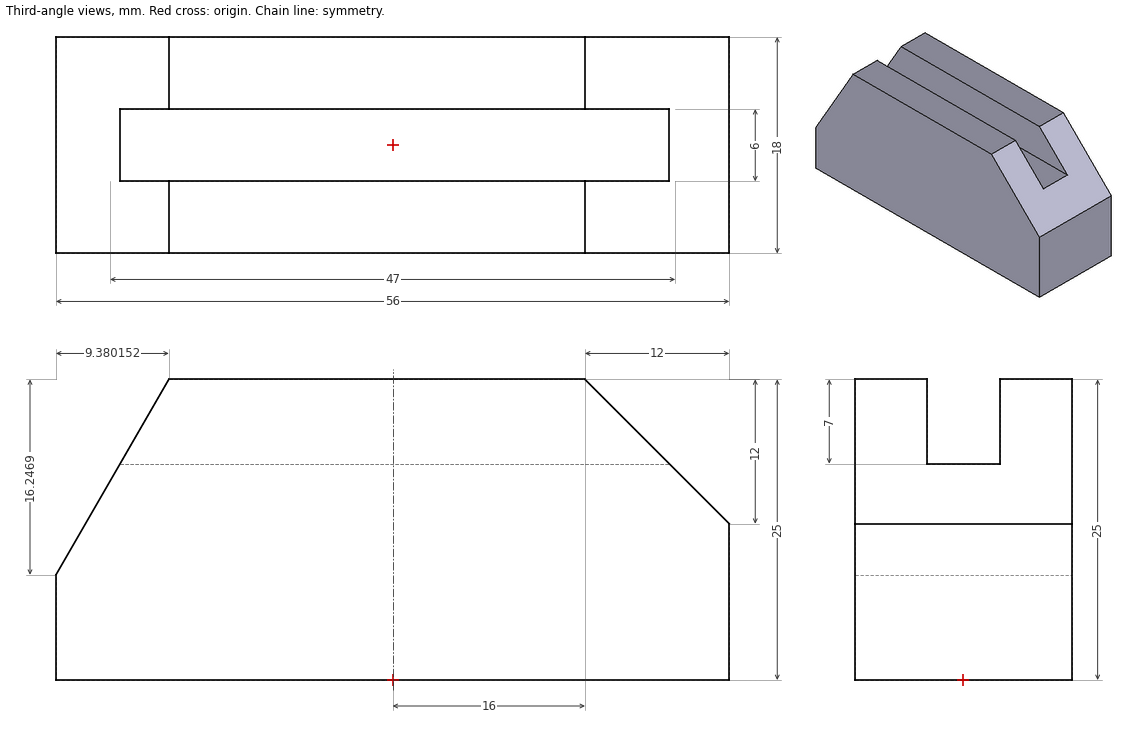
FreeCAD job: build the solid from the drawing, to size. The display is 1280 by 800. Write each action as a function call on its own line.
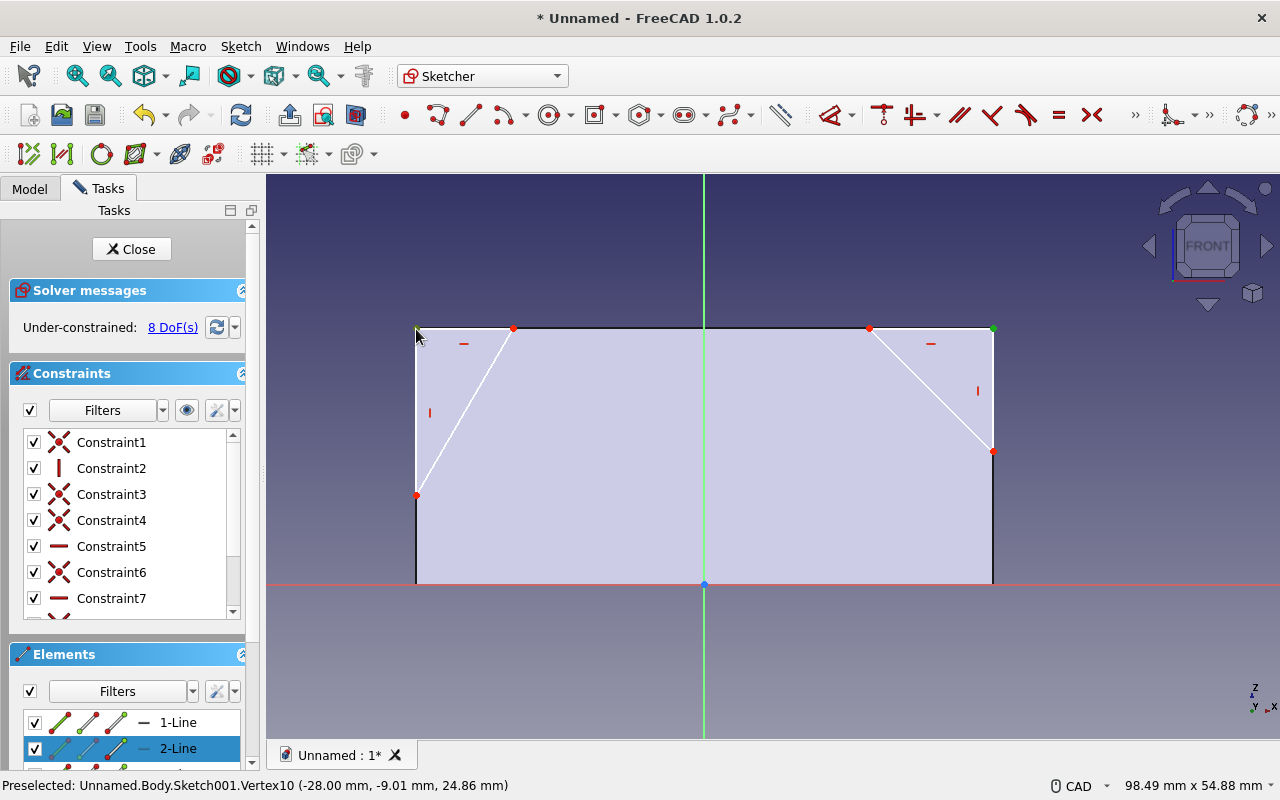
click(704, 675)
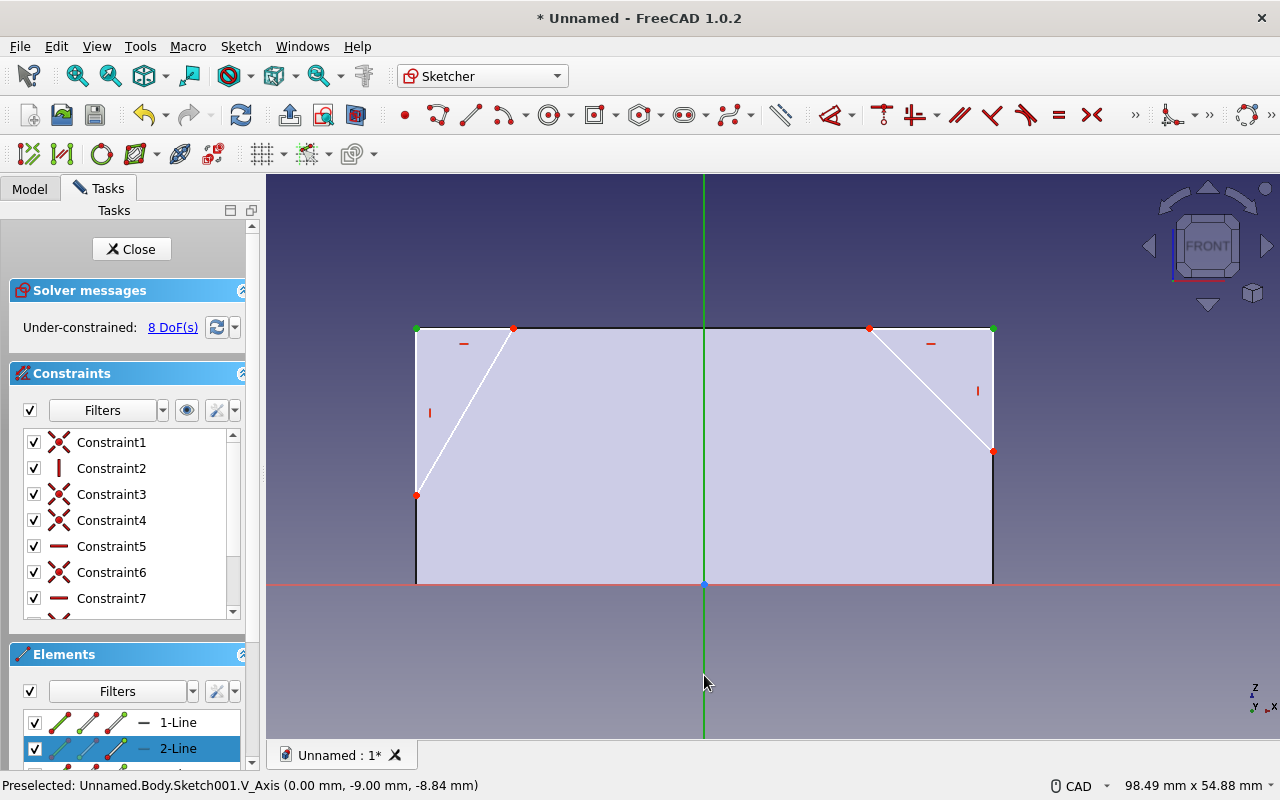
click(1092, 116)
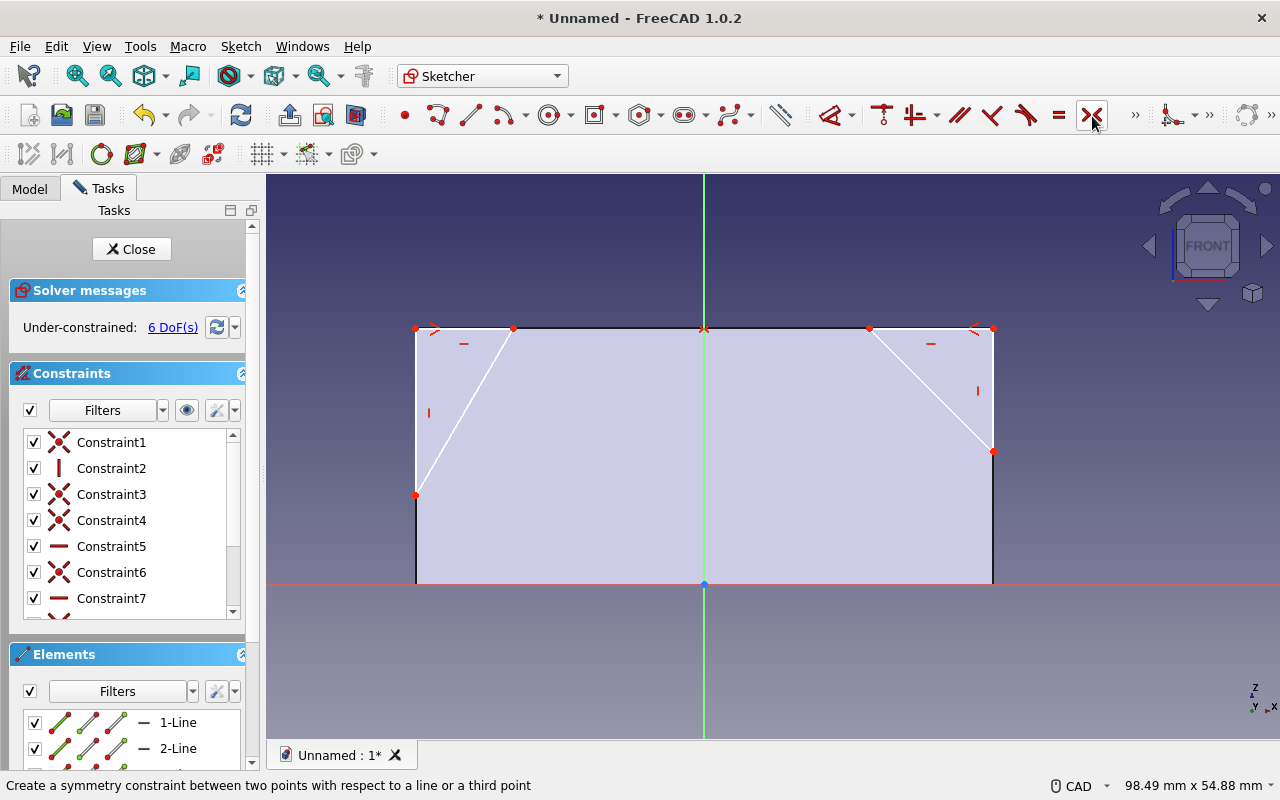
click(830, 116)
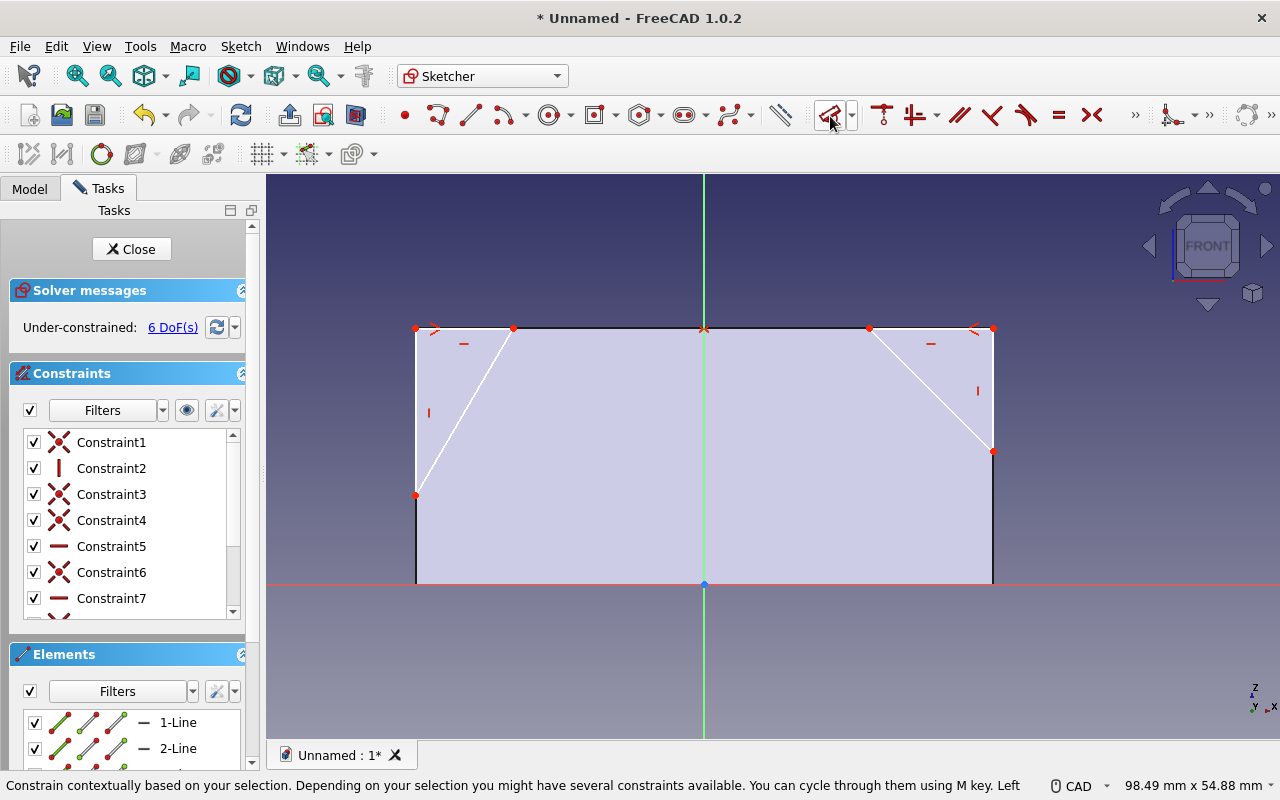
click(993, 415)
click(1027, 390)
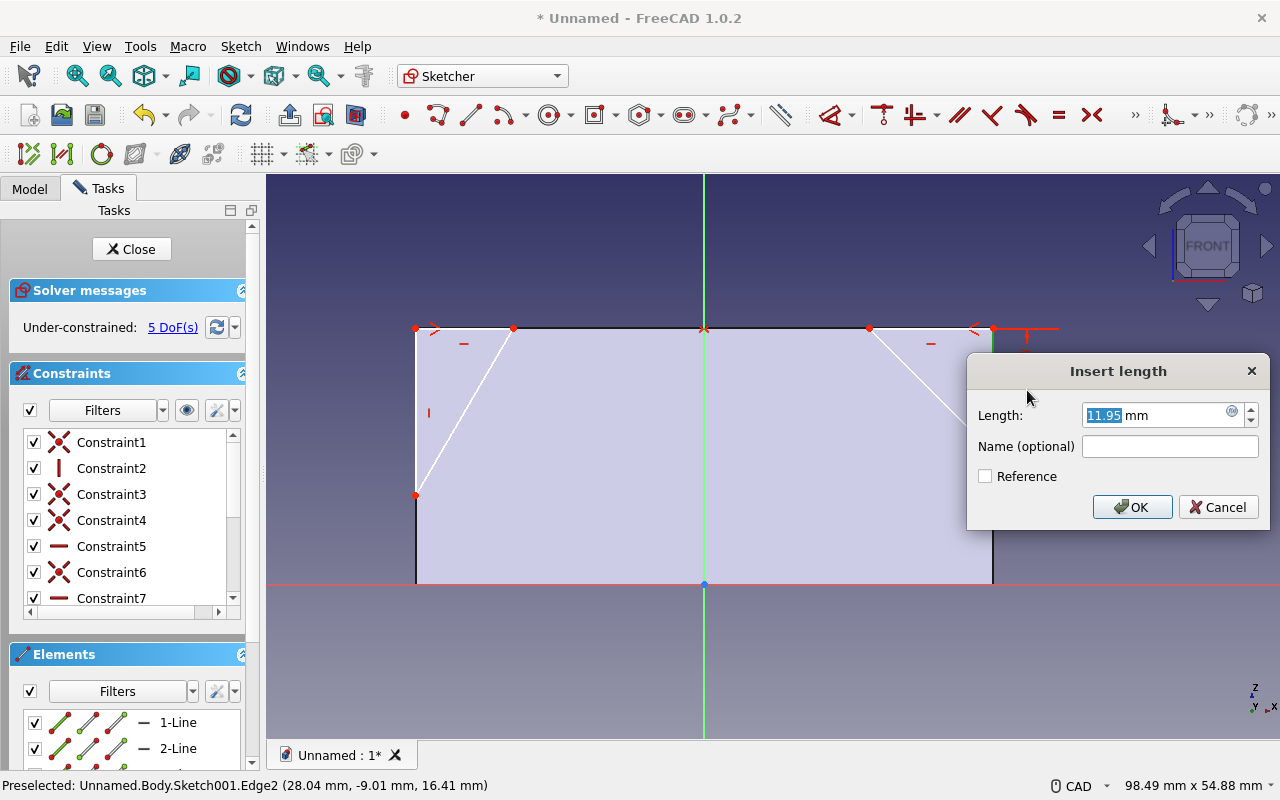
text(12)
key(Return)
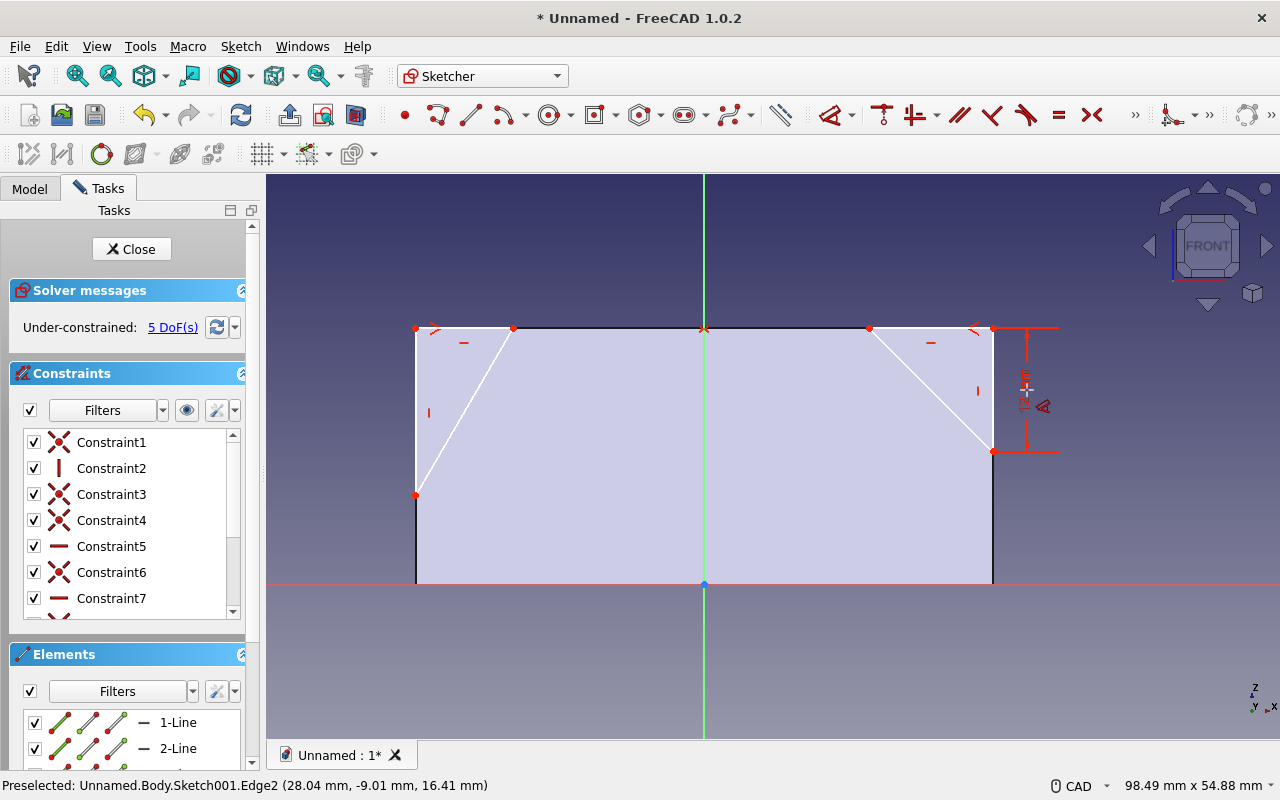
click(956, 328)
click(931, 294)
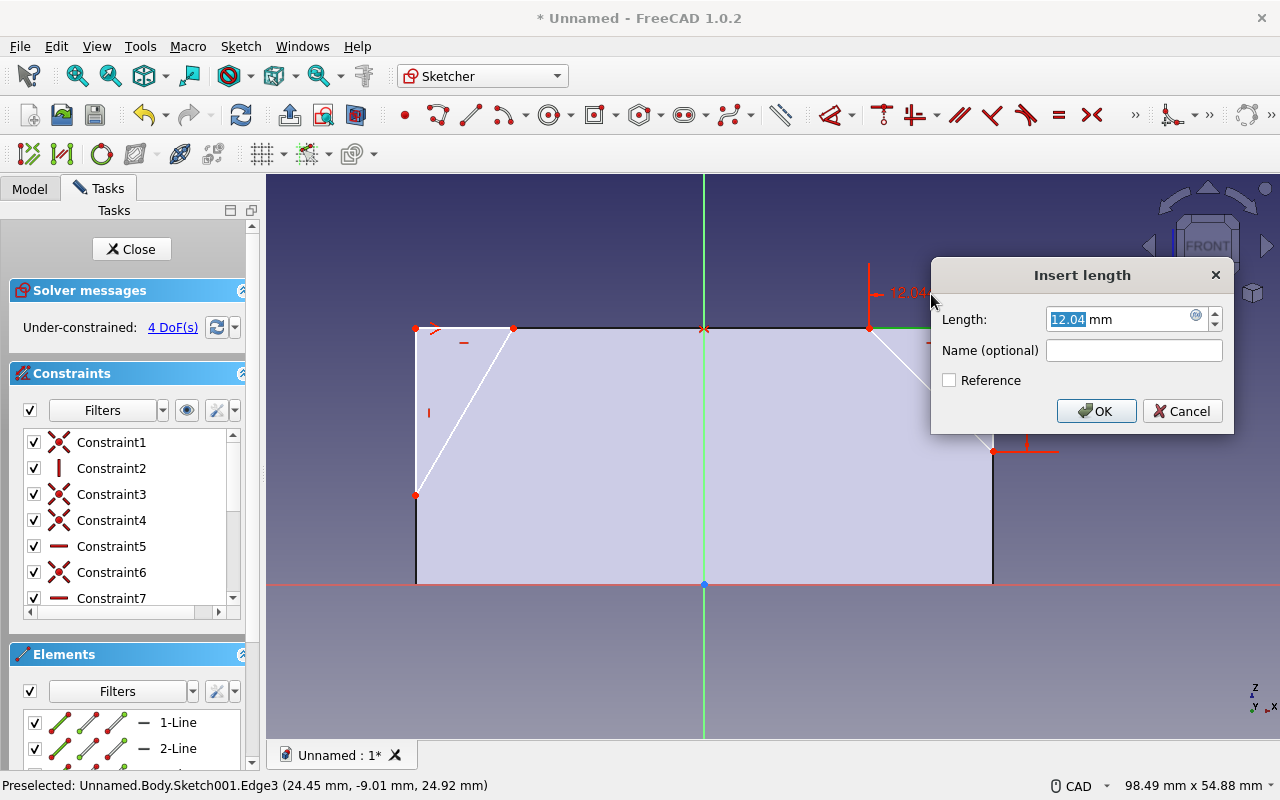
text(12)
key(Return)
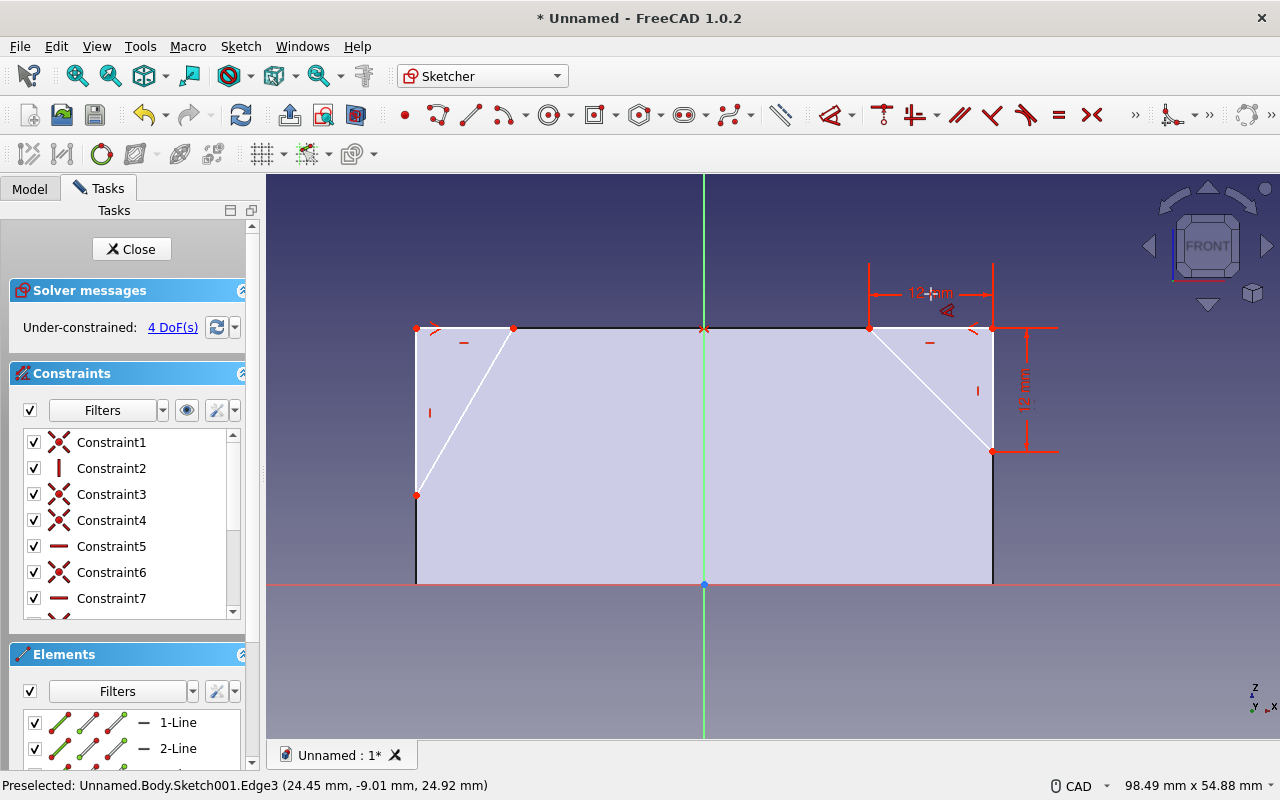
click(869, 328)
click(787, 619)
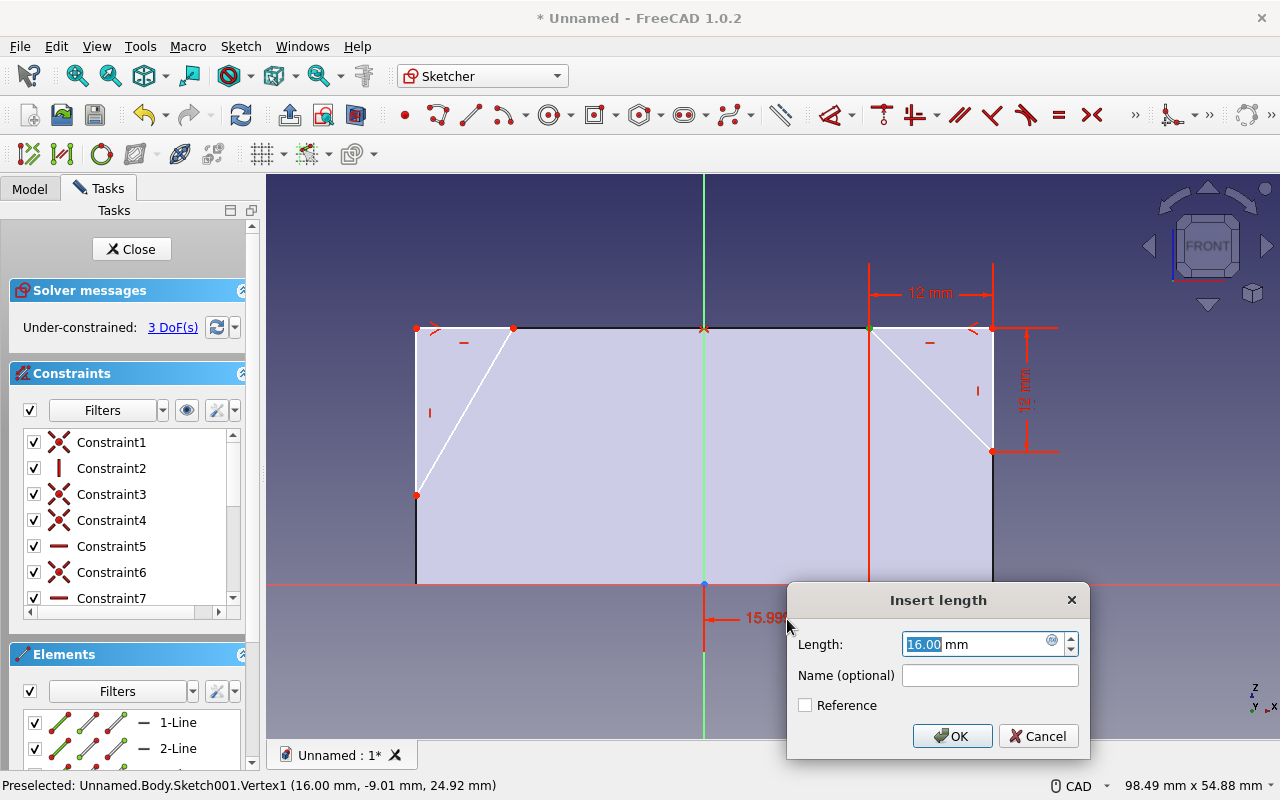
text(16)
key(Return)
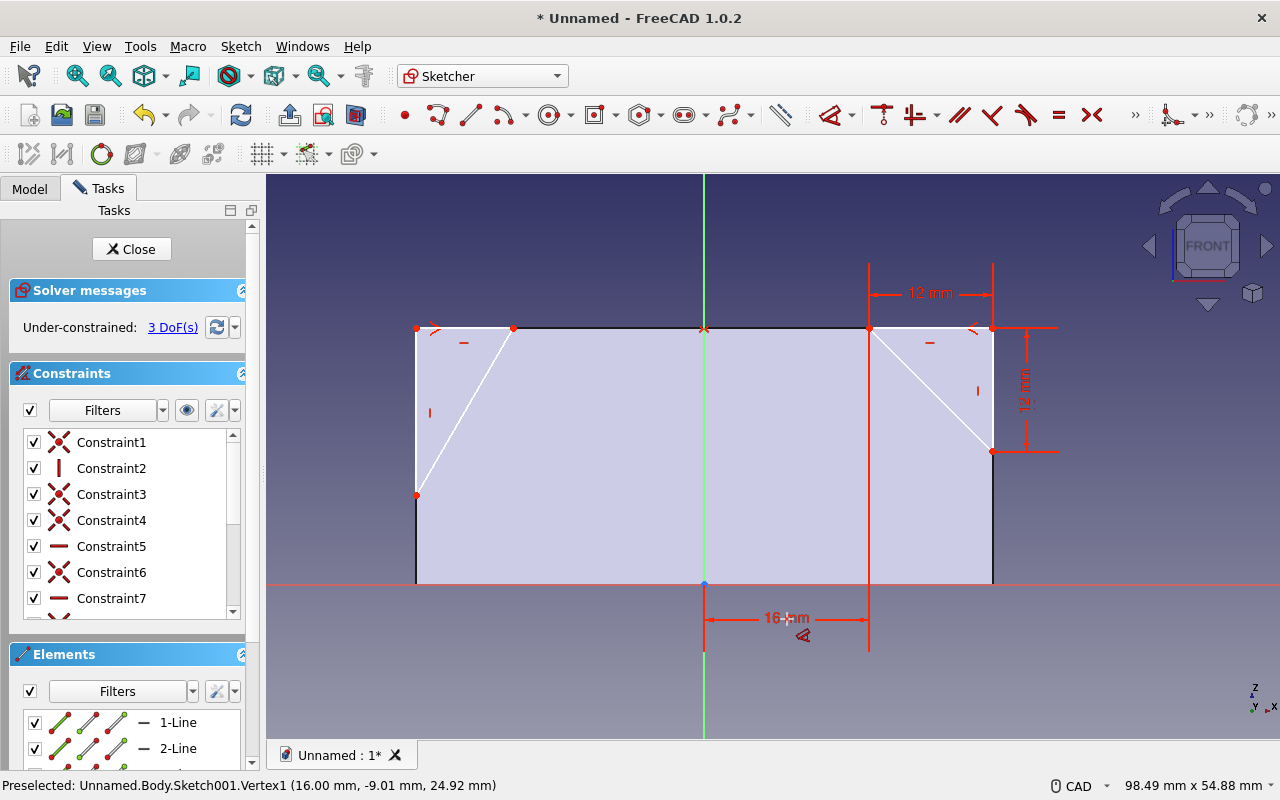
click(869, 328)
click(903, 457)